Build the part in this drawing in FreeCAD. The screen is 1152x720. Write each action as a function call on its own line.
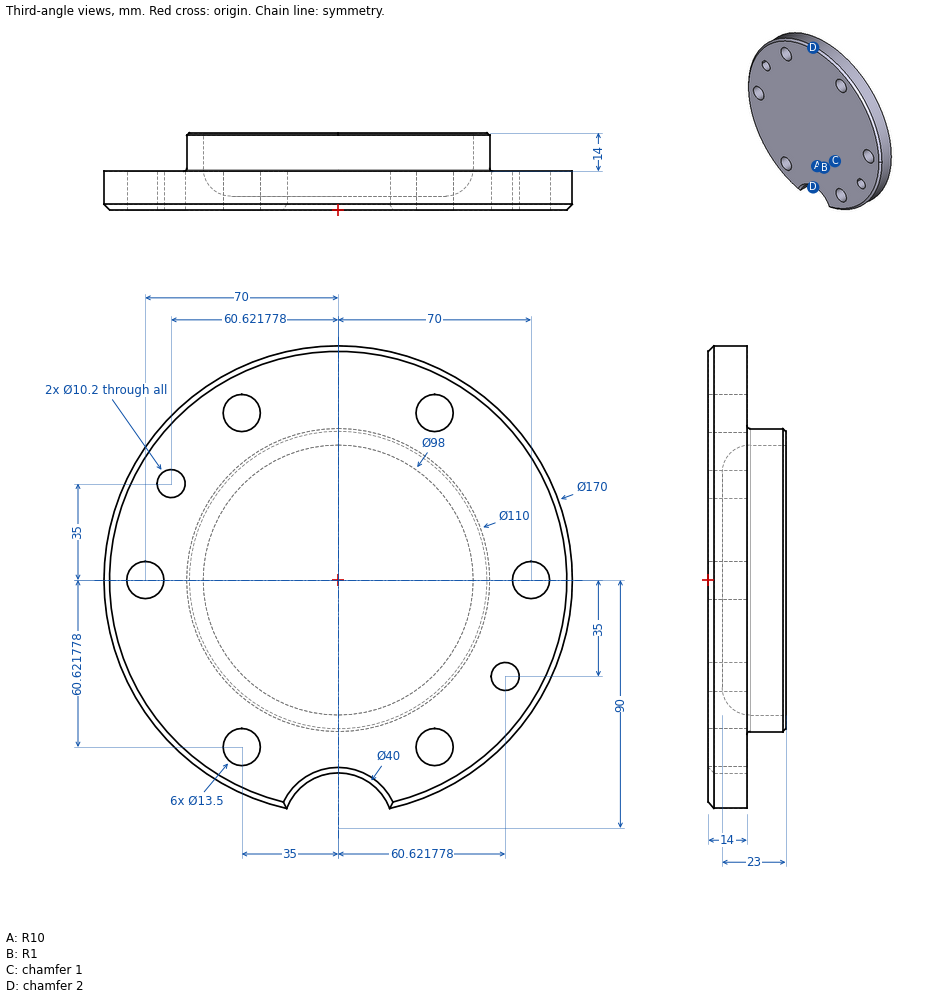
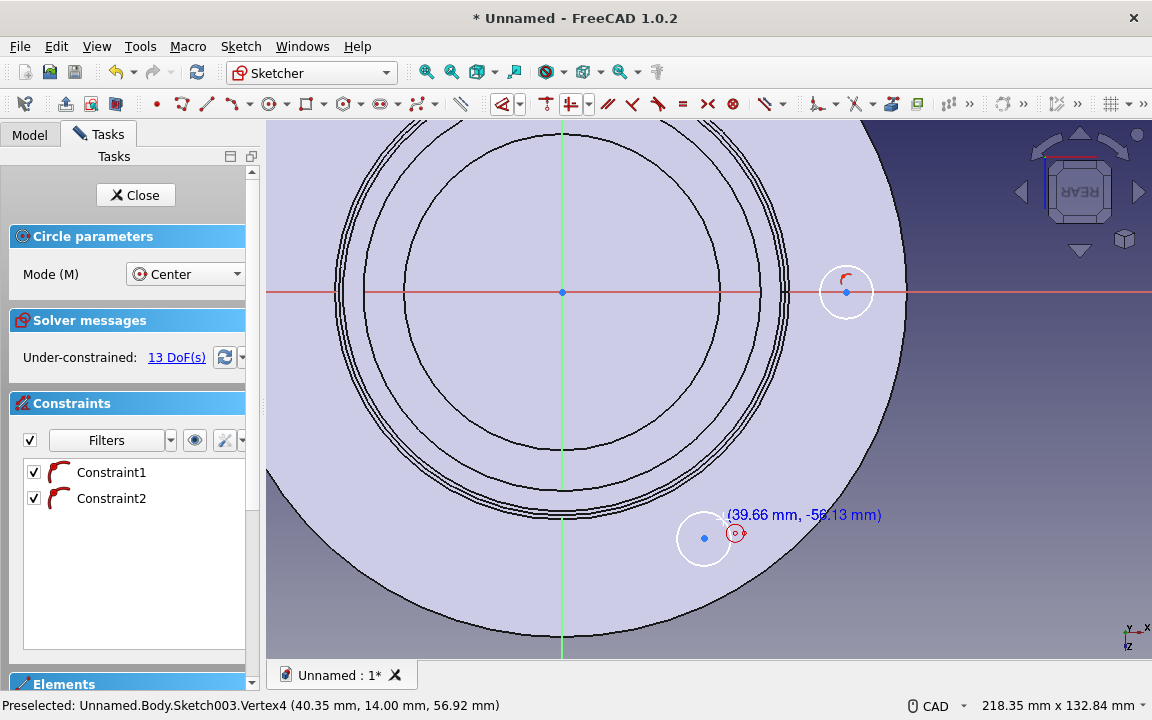
click(420, 538)
click(439, 519)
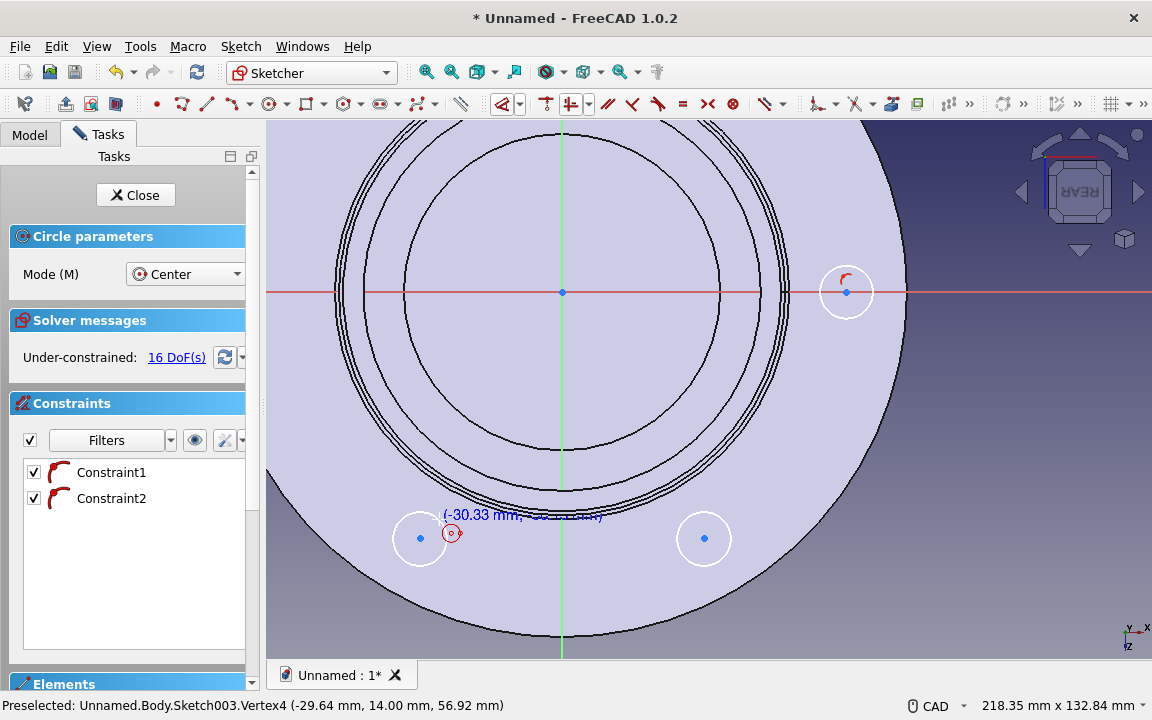
scroll(705, 539, down, 4)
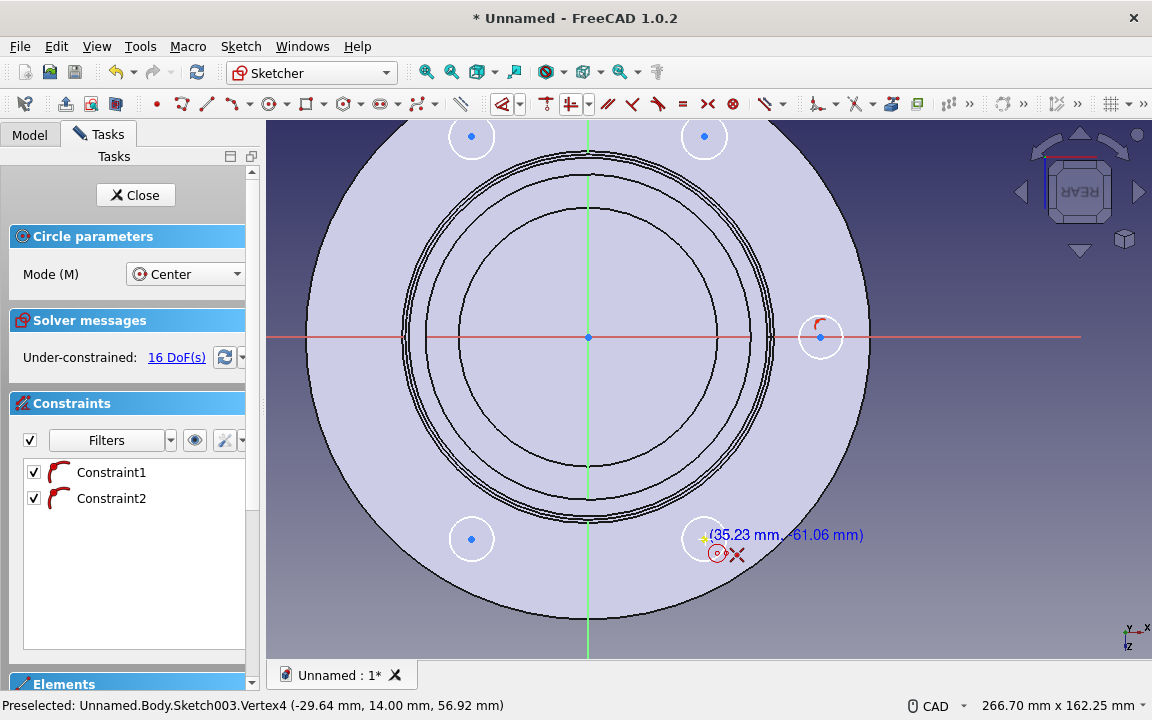
scroll(513, 429, up, 4)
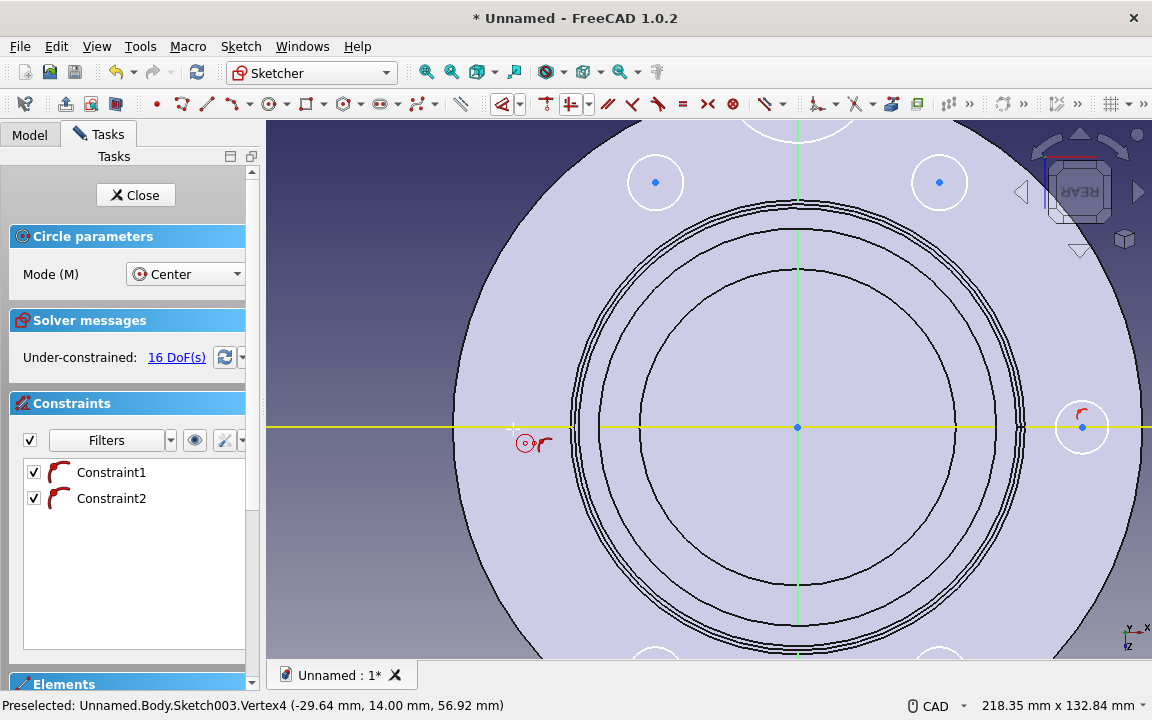
click(514, 427)
click(533, 408)
key(Escape)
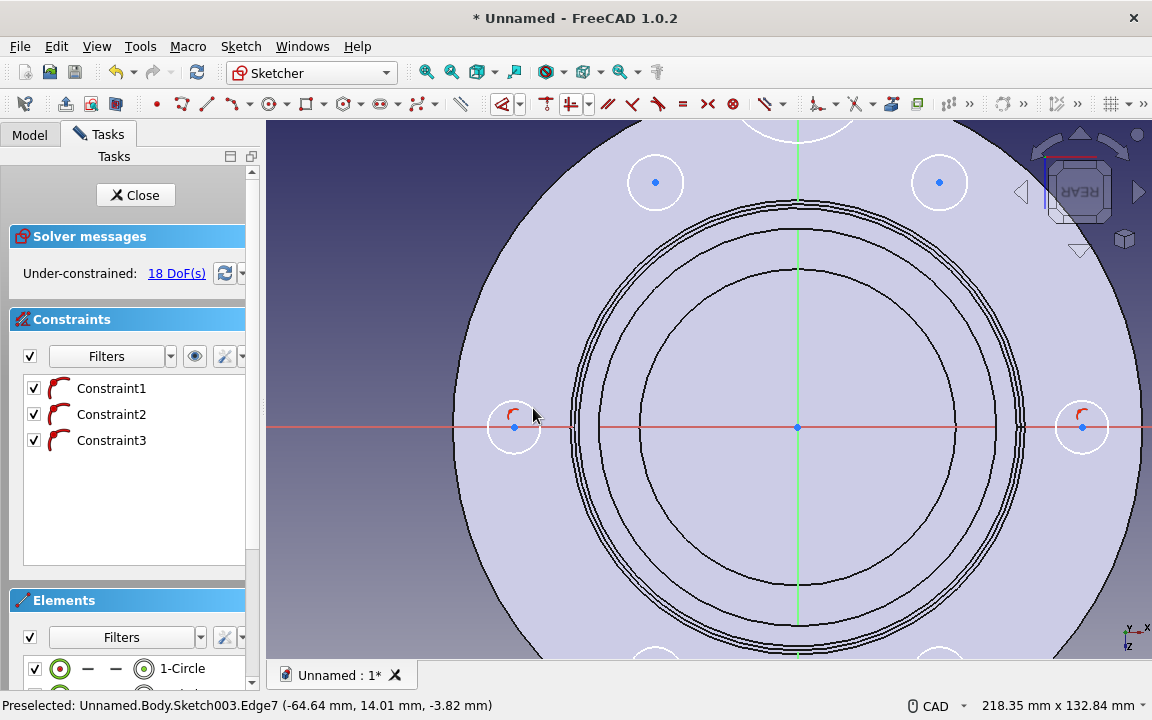
click(675, 163)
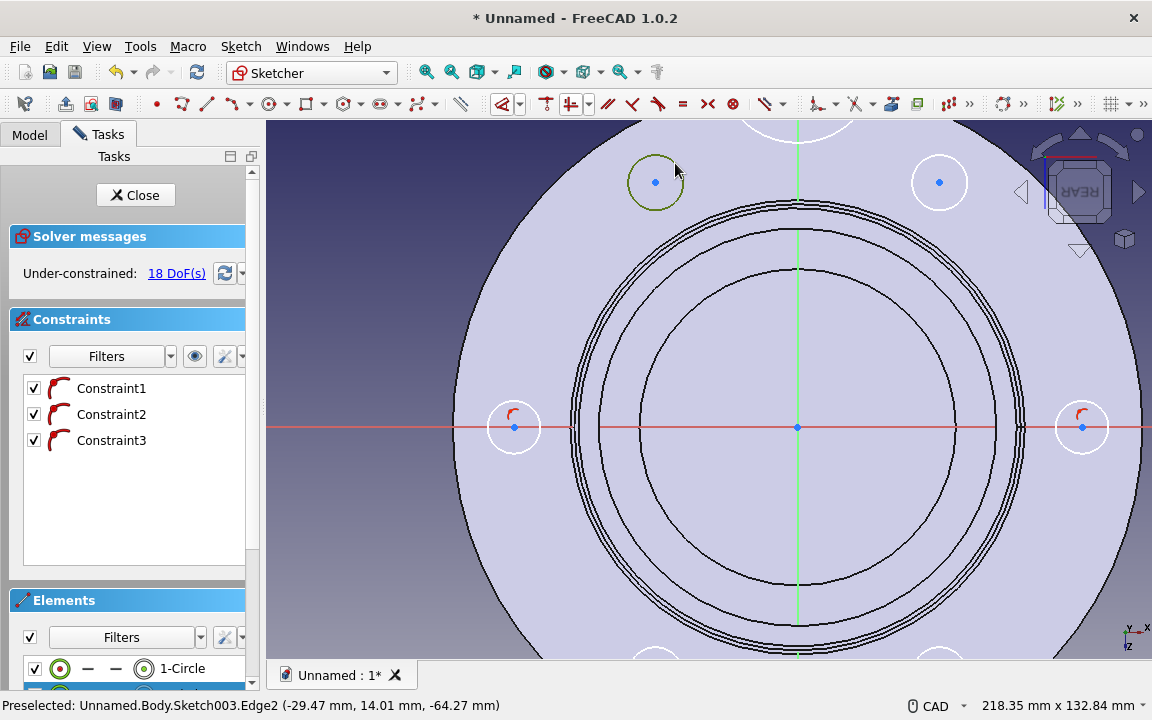
click(959, 163)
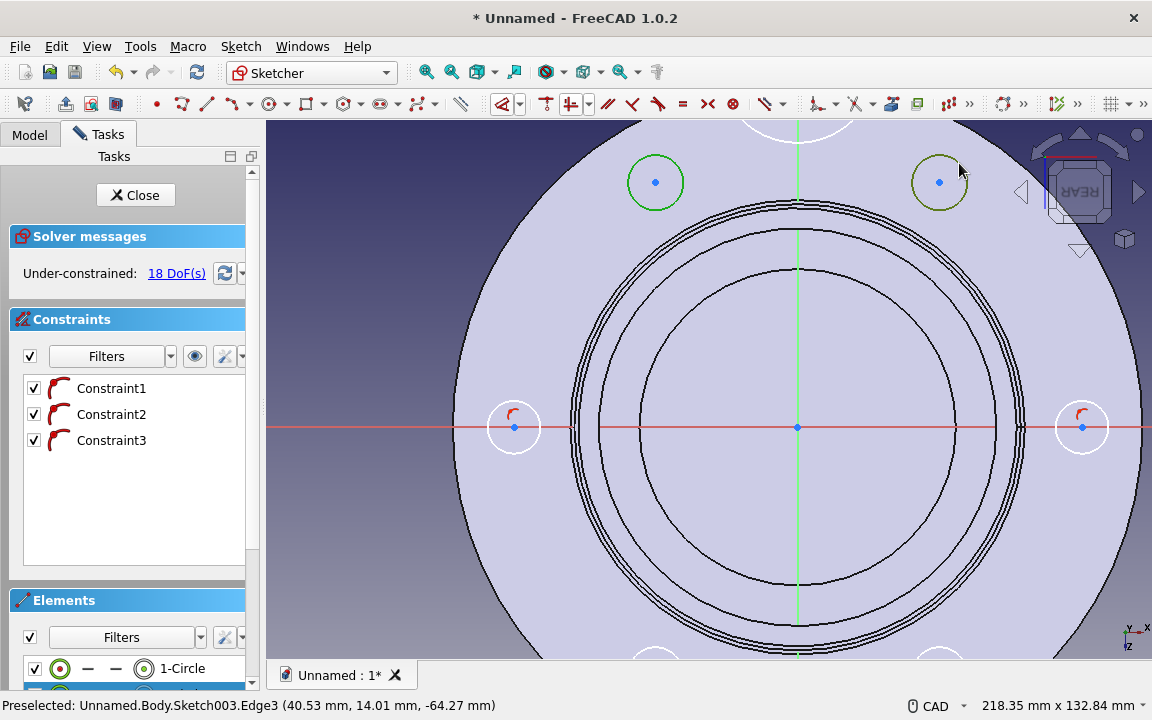
scroll(512, 429, down, 4)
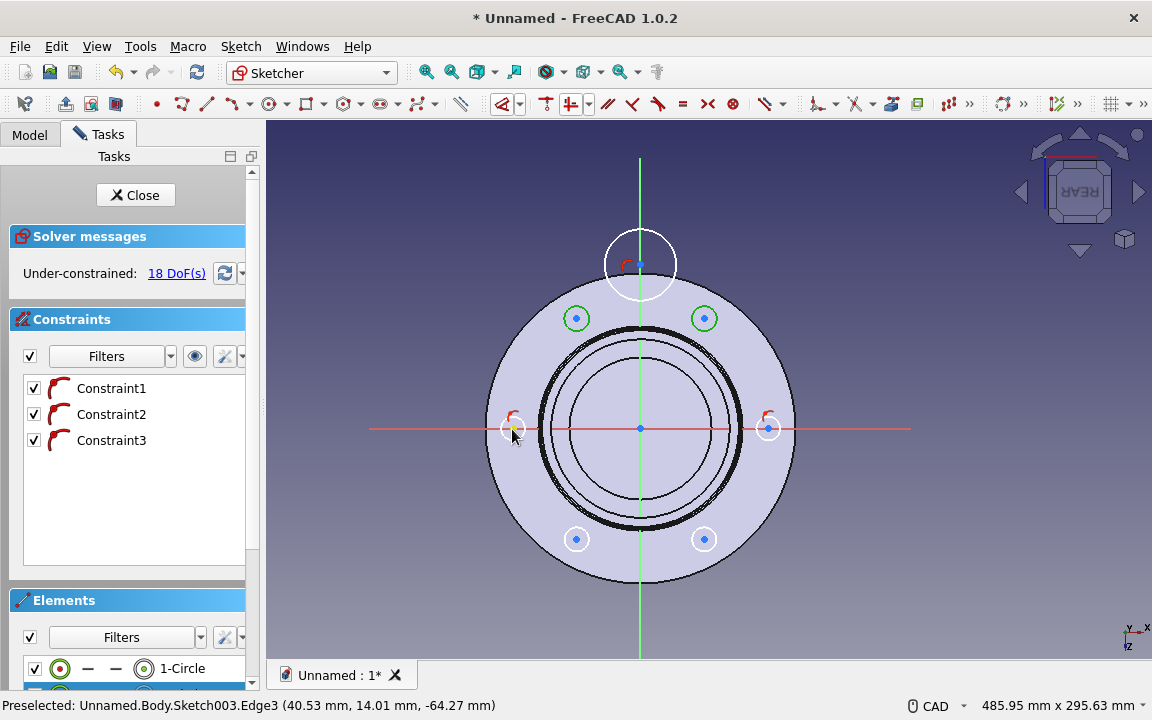
scroll(777, 420, up, 3)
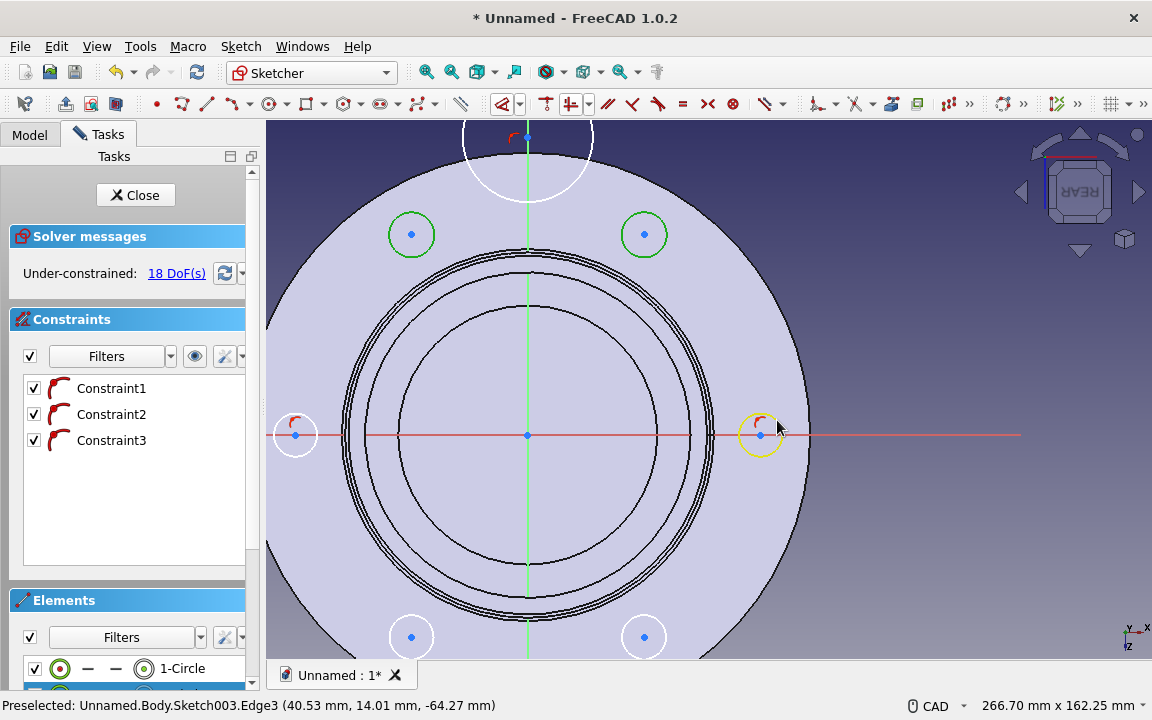
click(776, 420)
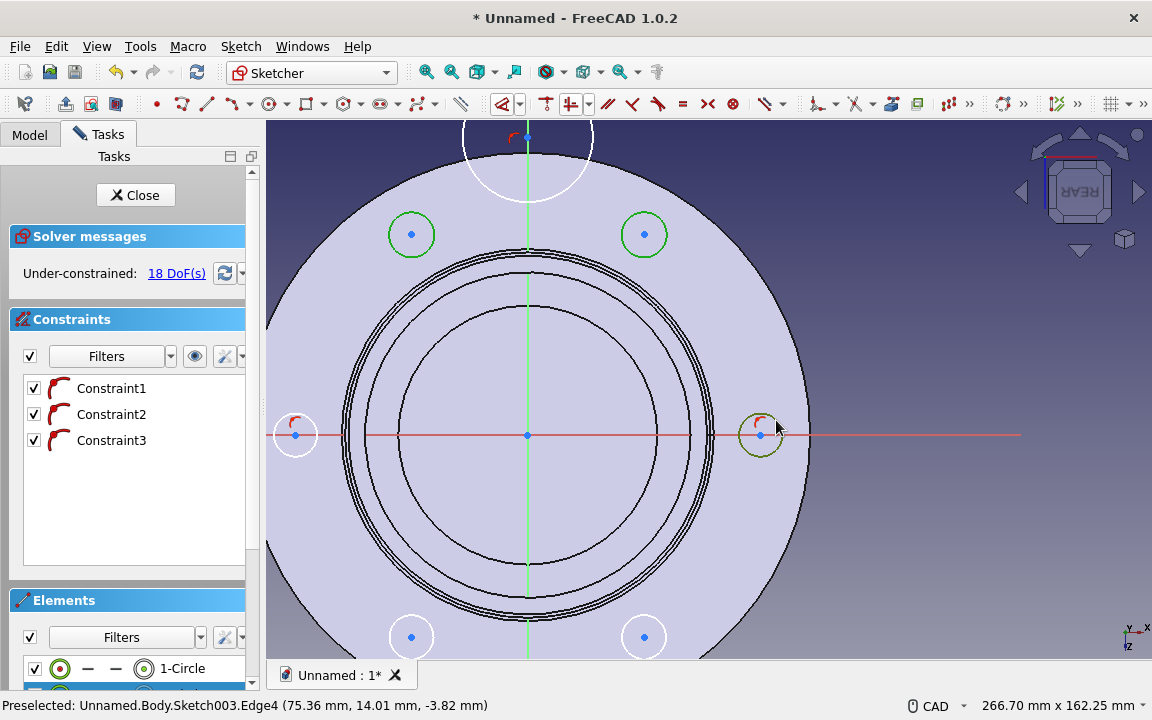
click(660, 622)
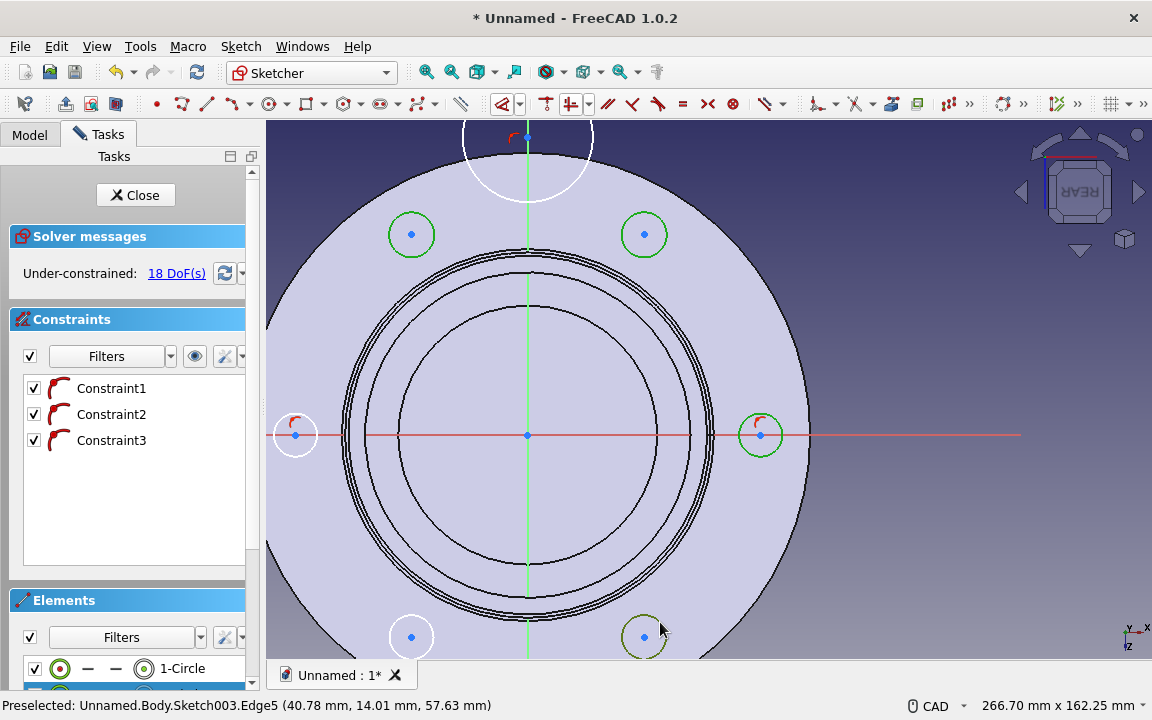
click(427, 622)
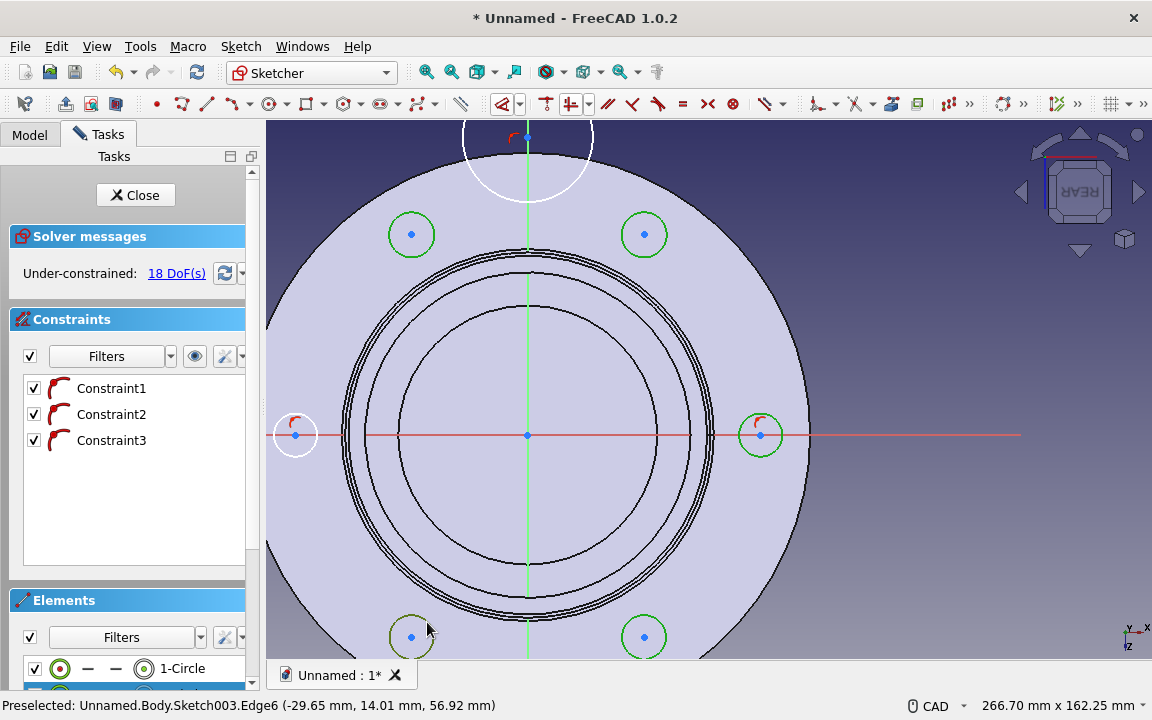
click(311, 420)